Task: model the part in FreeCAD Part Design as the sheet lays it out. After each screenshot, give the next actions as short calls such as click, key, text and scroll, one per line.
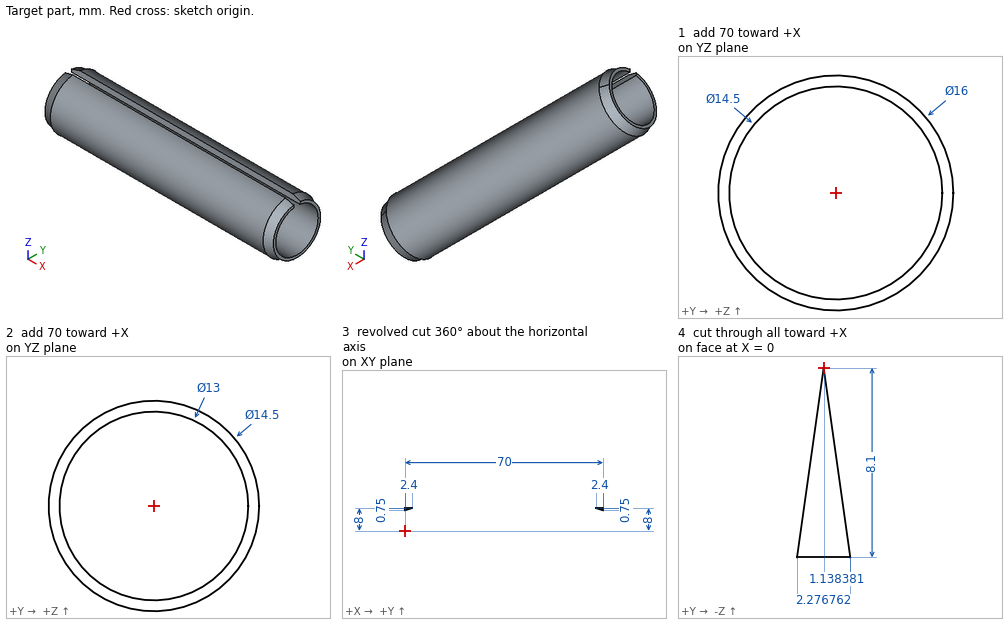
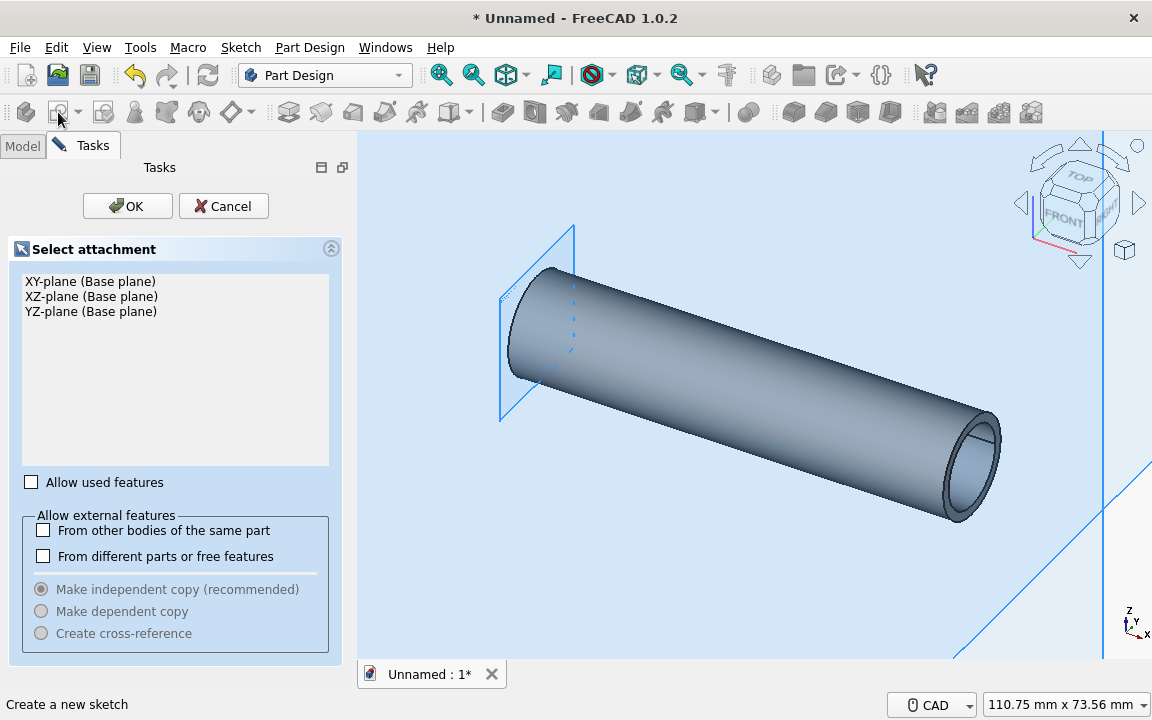
click(82, 282)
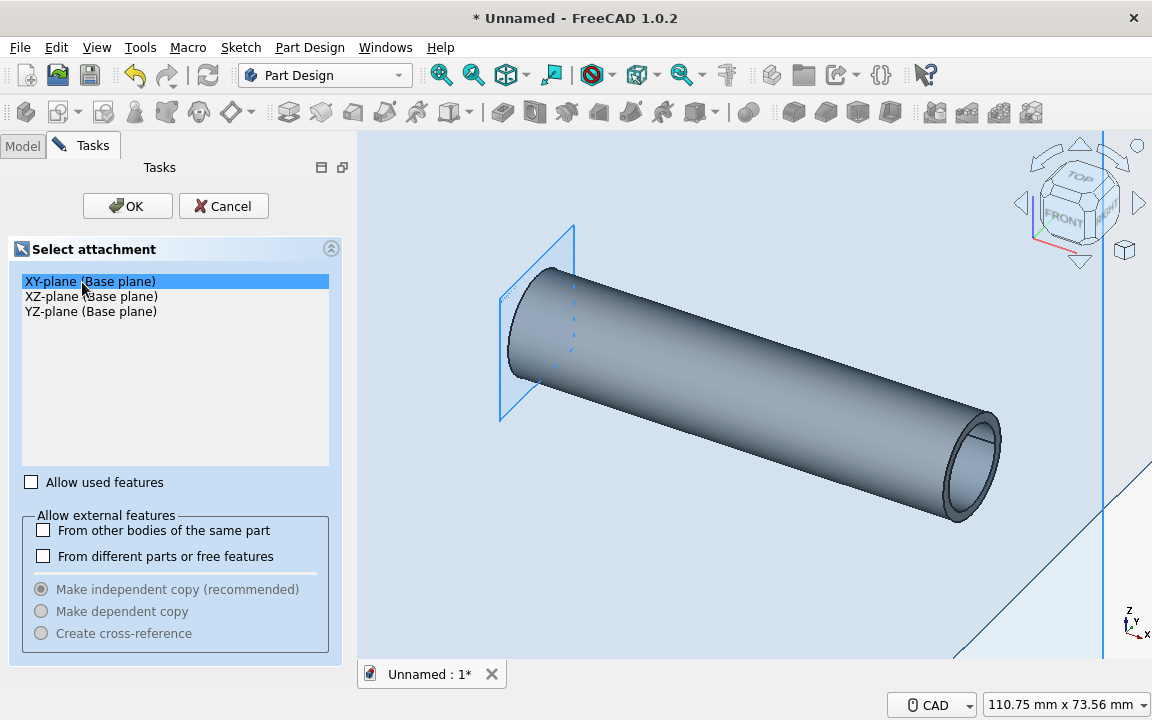
click(128, 206)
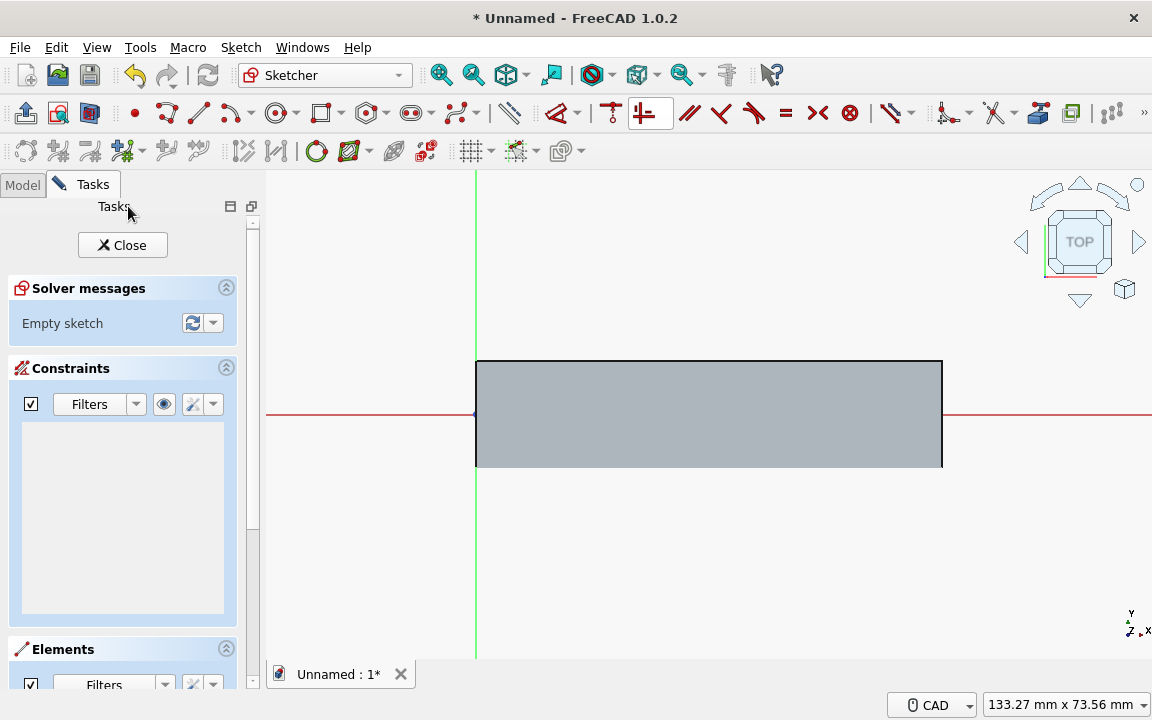
click(90, 114)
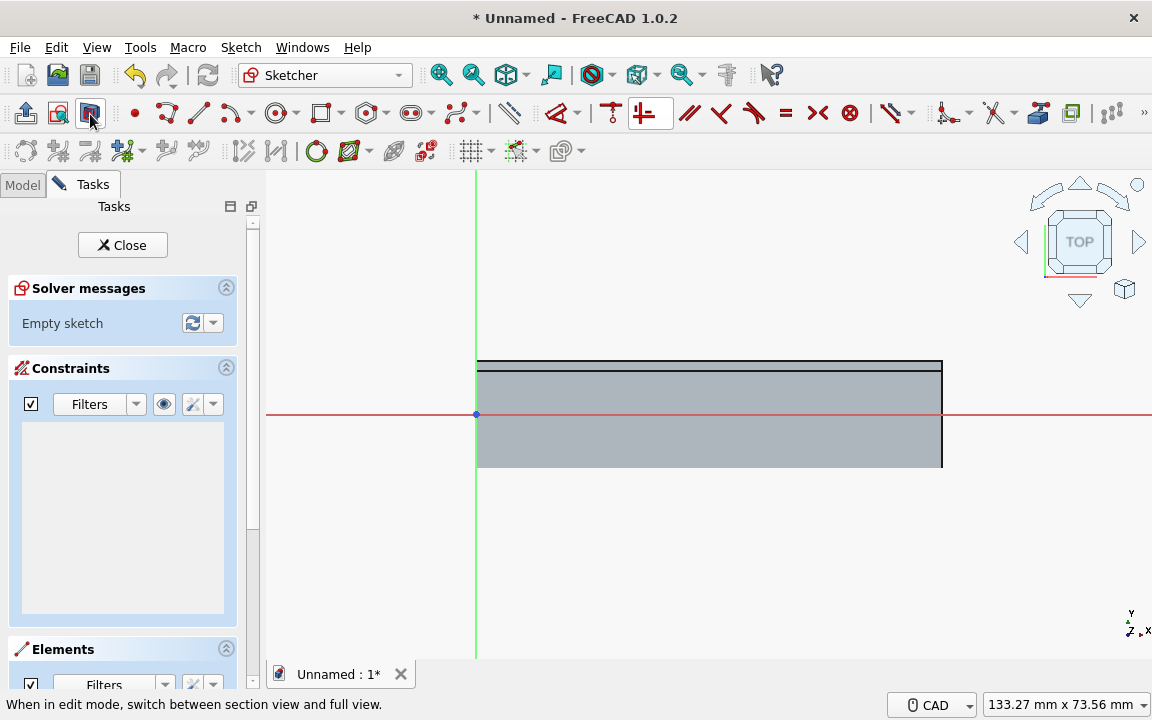
click(168, 114)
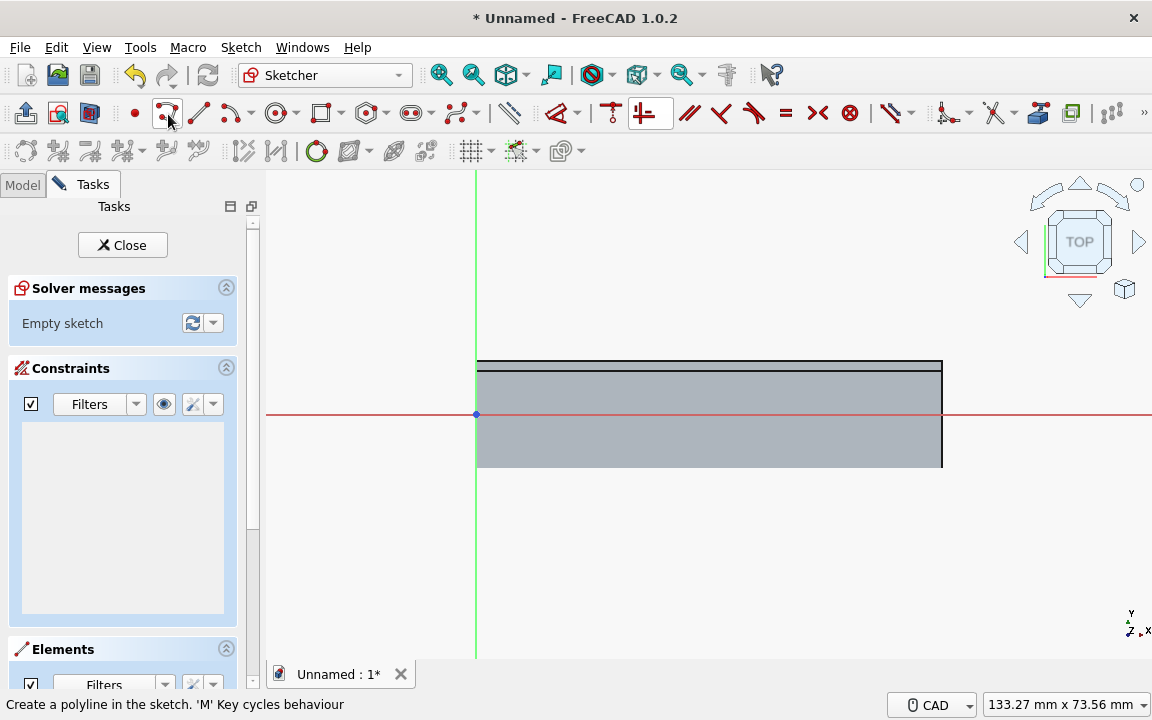
click(926, 361)
click(942, 366)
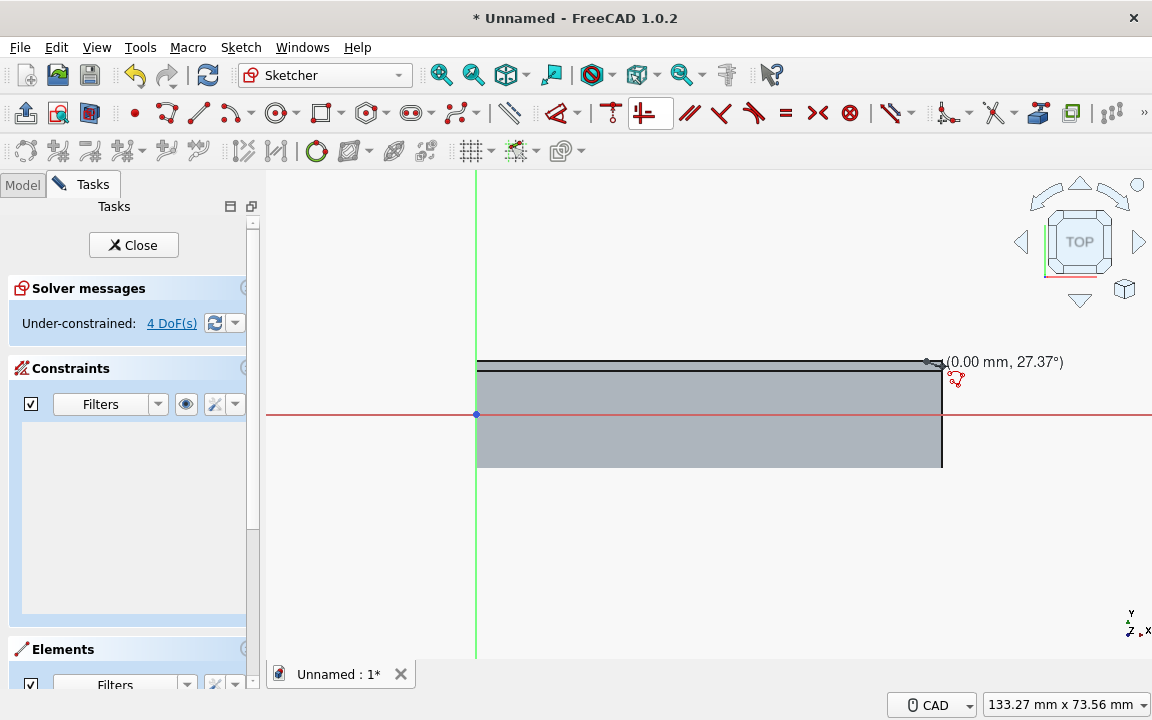
scroll(942, 361, up, 7)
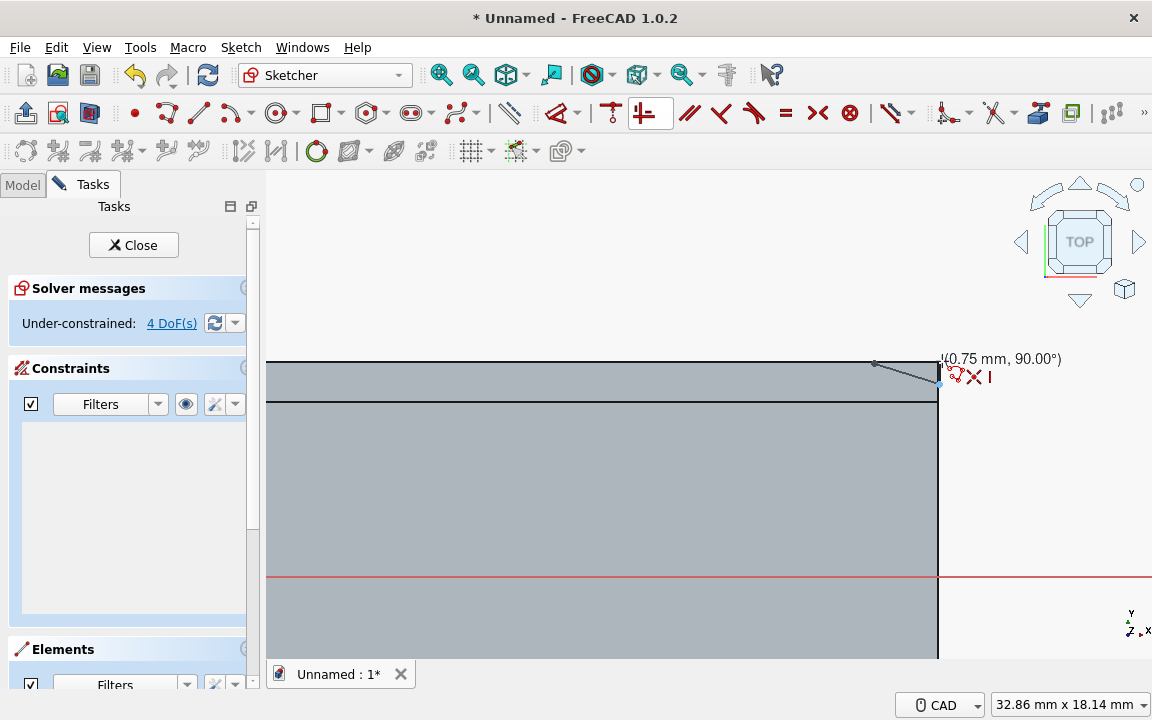
click(940, 362)
click(875, 364)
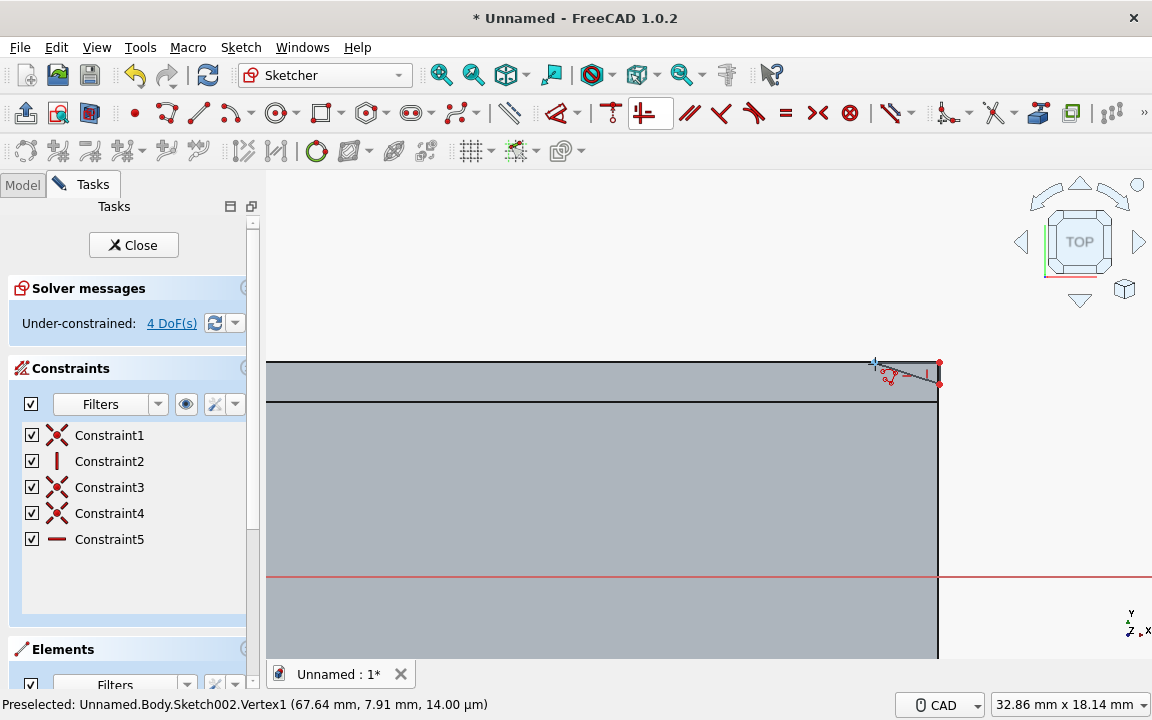
scroll(852, 397, down, 7)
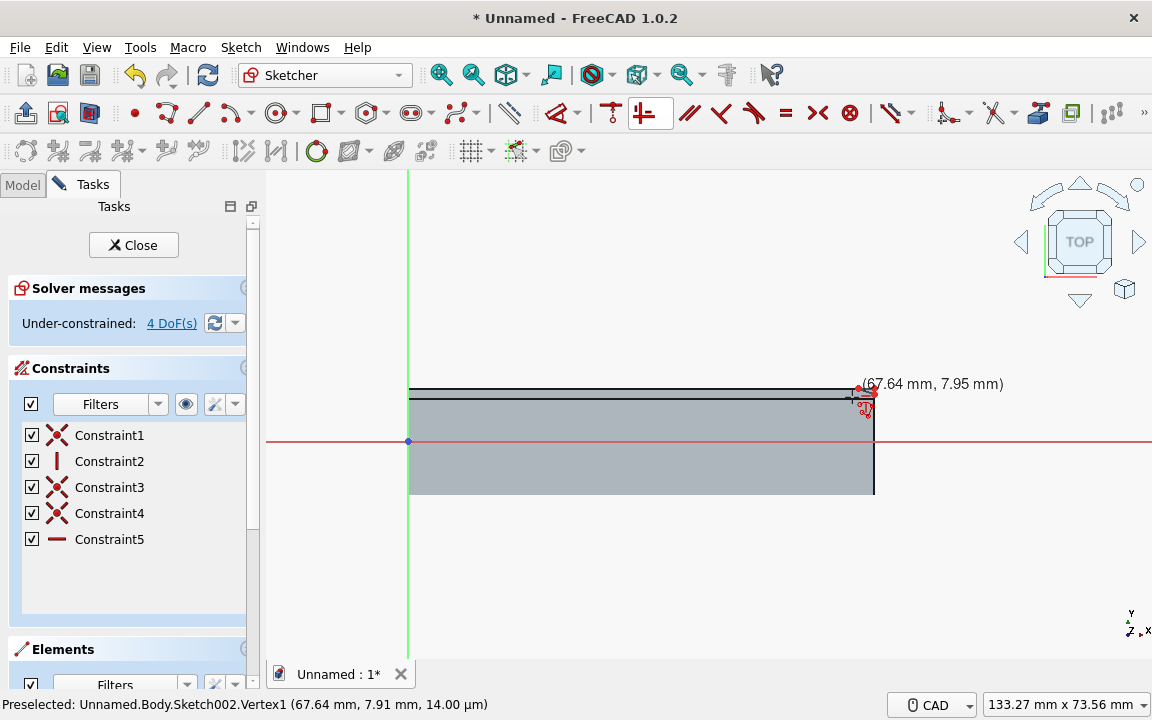
click(408, 394)
click(424, 389)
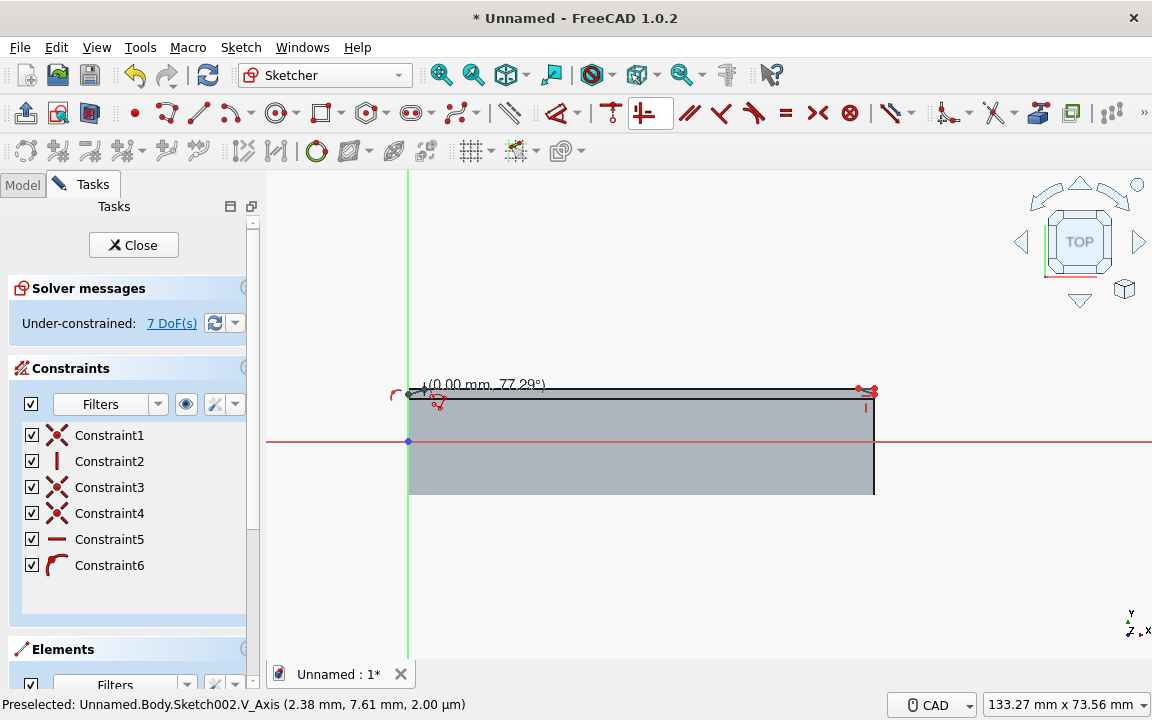
scroll(408, 389, up, 7)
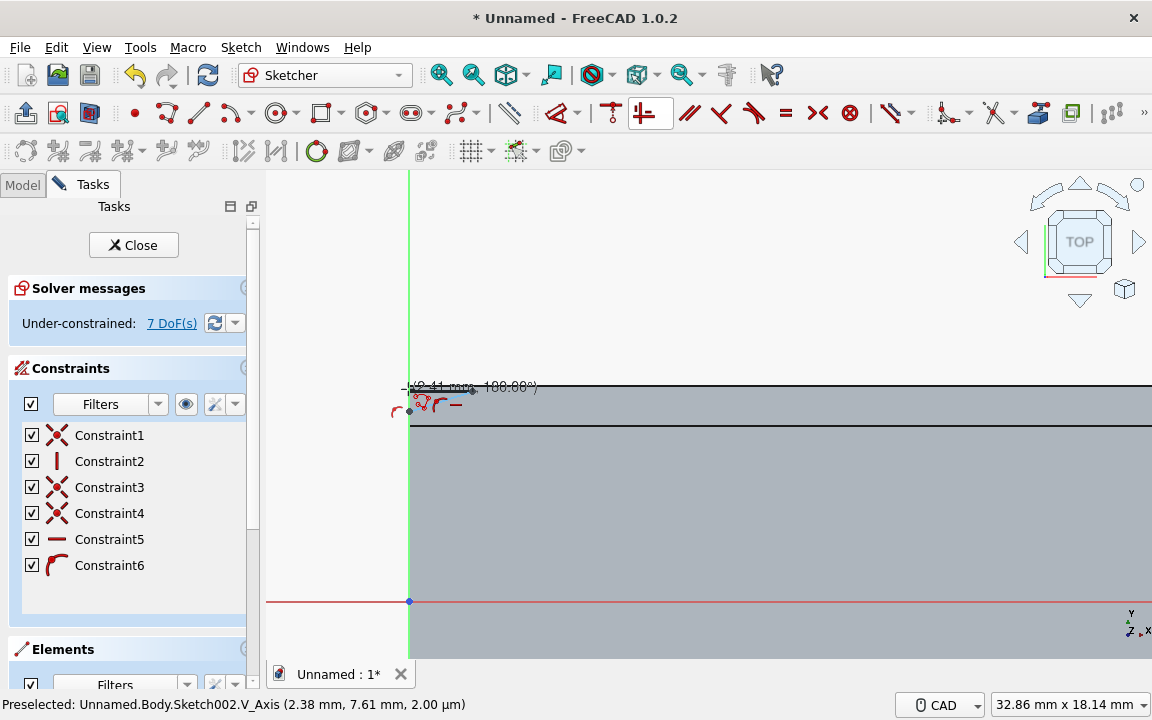
click(418, 388)
click(409, 412)
key(Escape)
key(Escape)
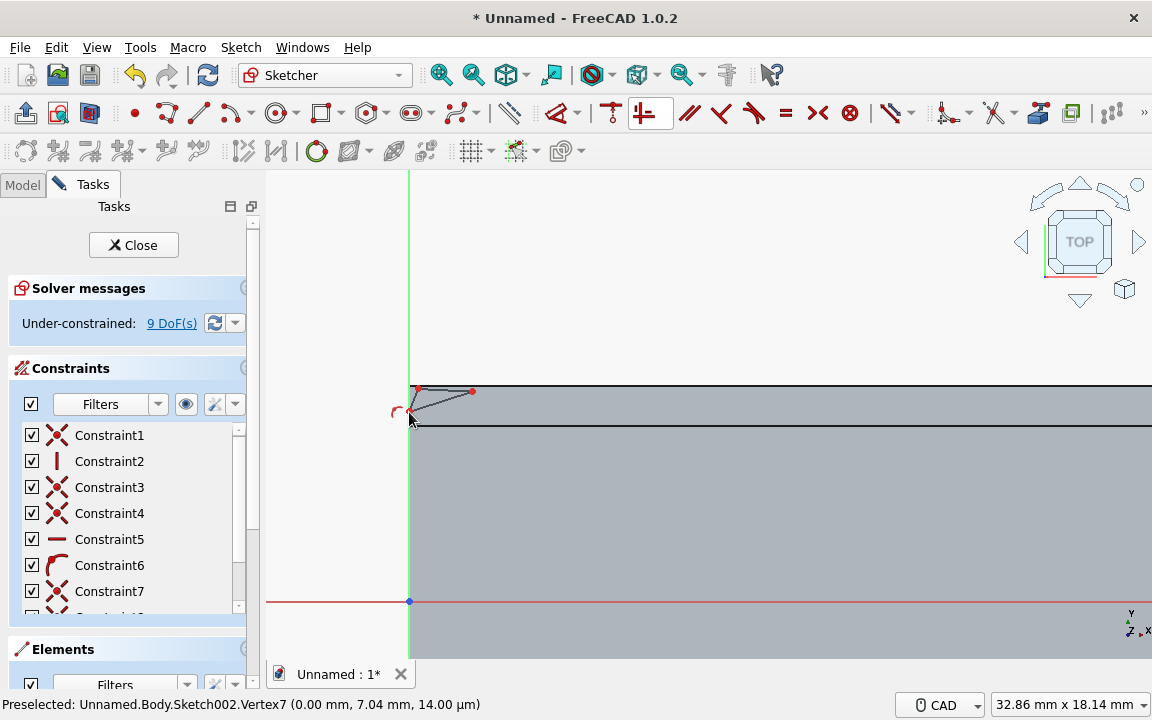
click(434, 390)